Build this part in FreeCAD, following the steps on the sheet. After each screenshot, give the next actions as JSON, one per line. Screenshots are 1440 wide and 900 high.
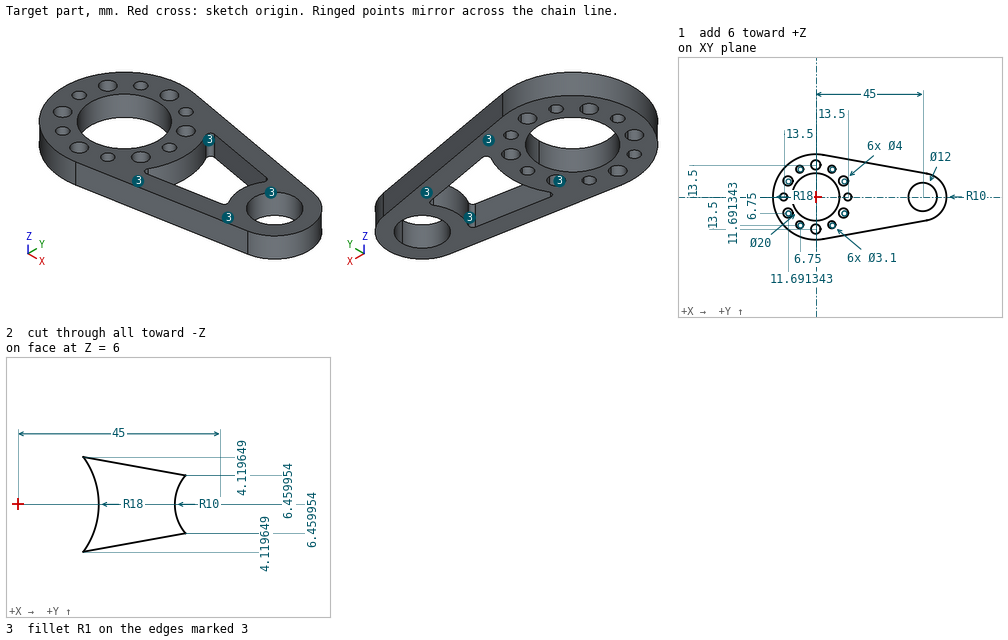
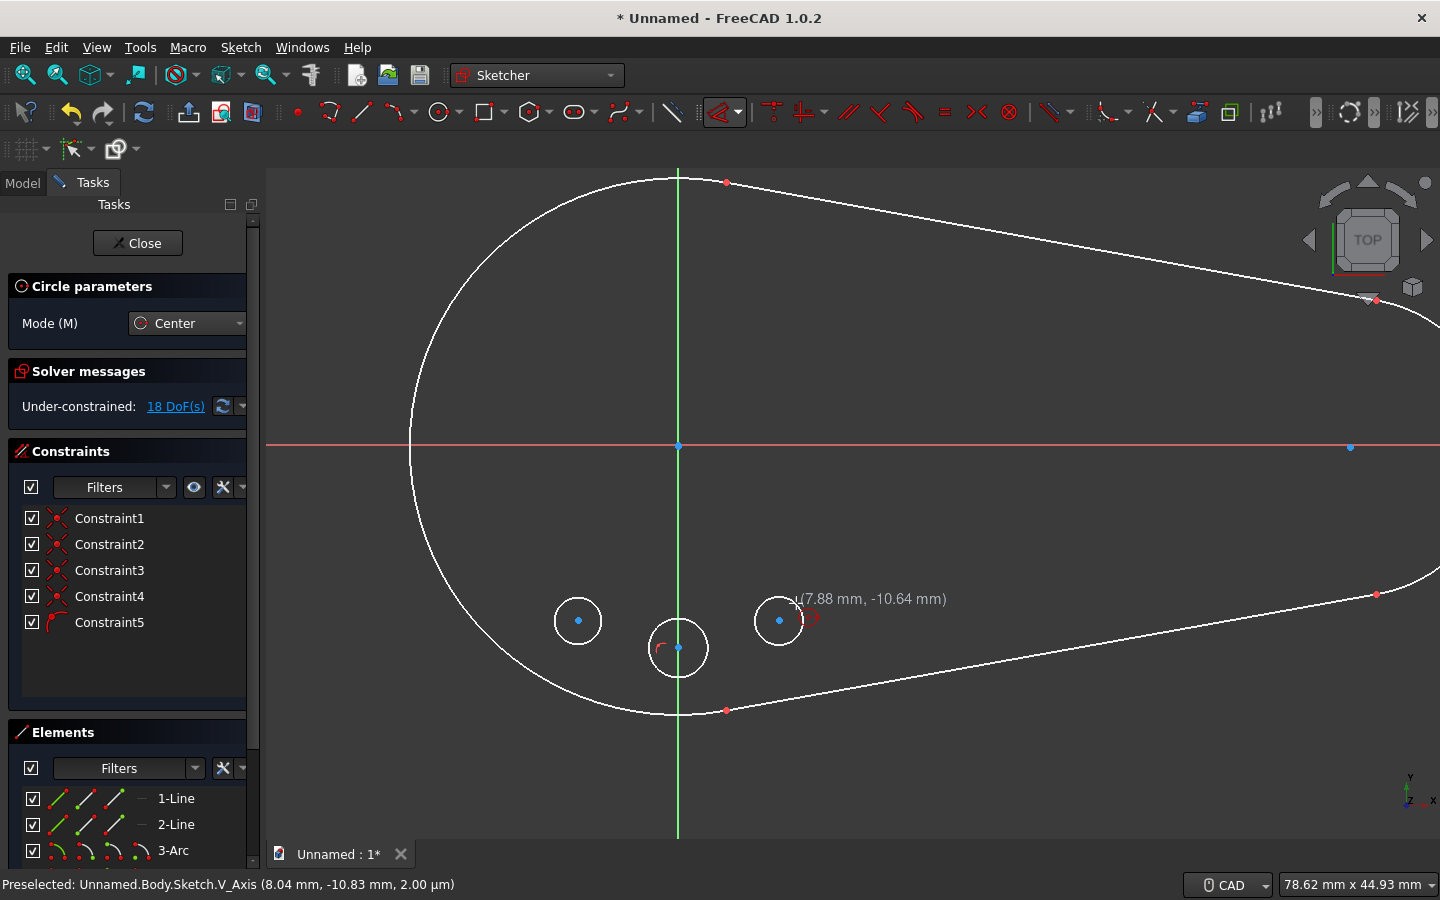
{"action": "left_click", "coordinate": [504, 546]}
{"action": "left_click", "coordinate": [525, 525]}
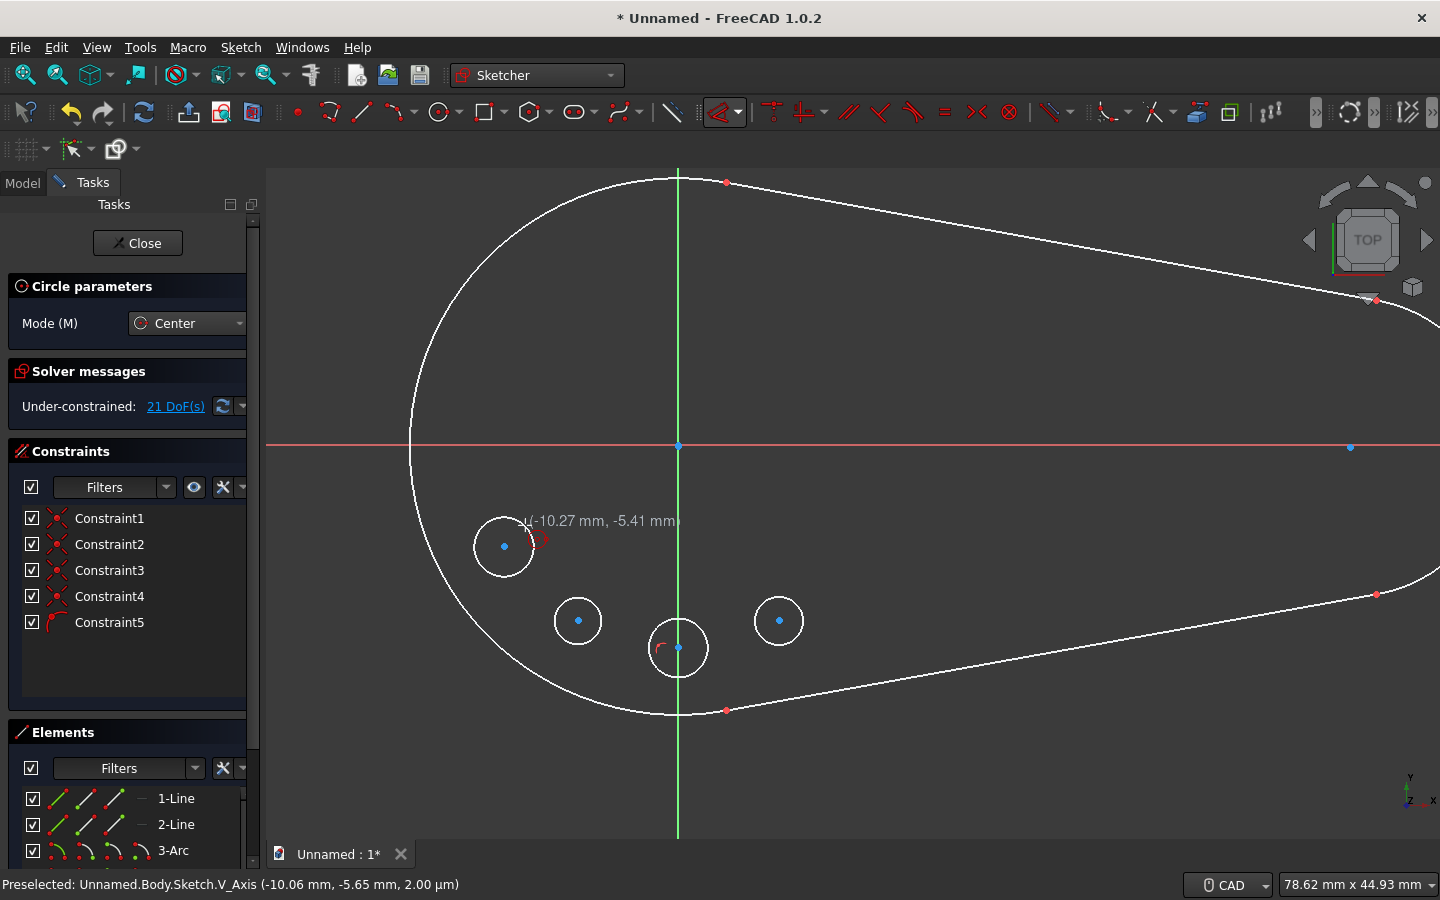
{"action": "left_click", "coordinate": [853, 546]}
{"action": "left_click", "coordinate": [874, 525]}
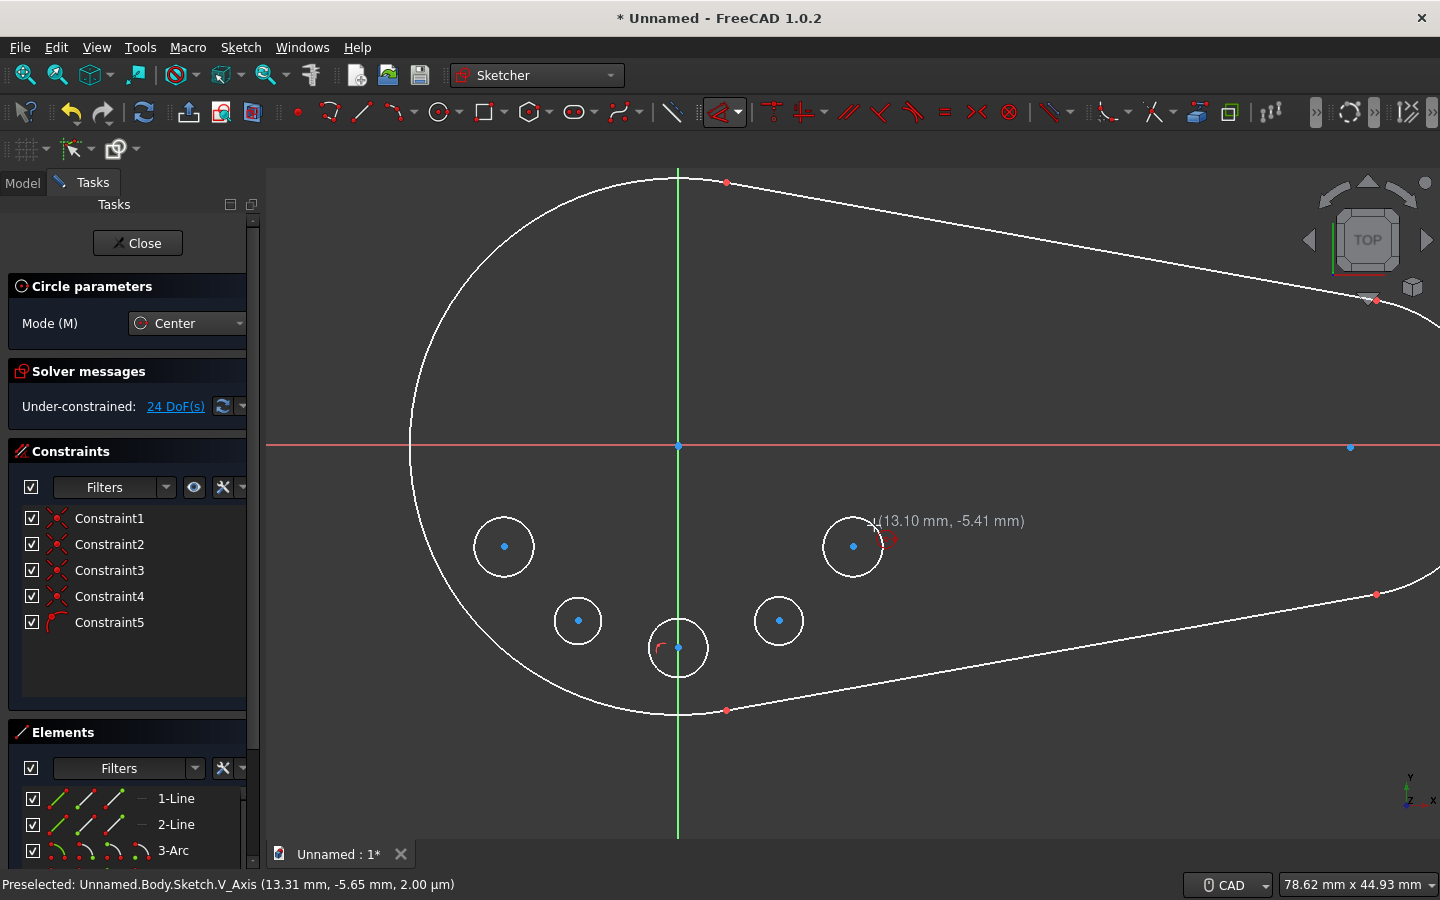
{"action": "left_click", "coordinate": [477, 445]}
{"action": "left_click", "coordinate": [493, 429]}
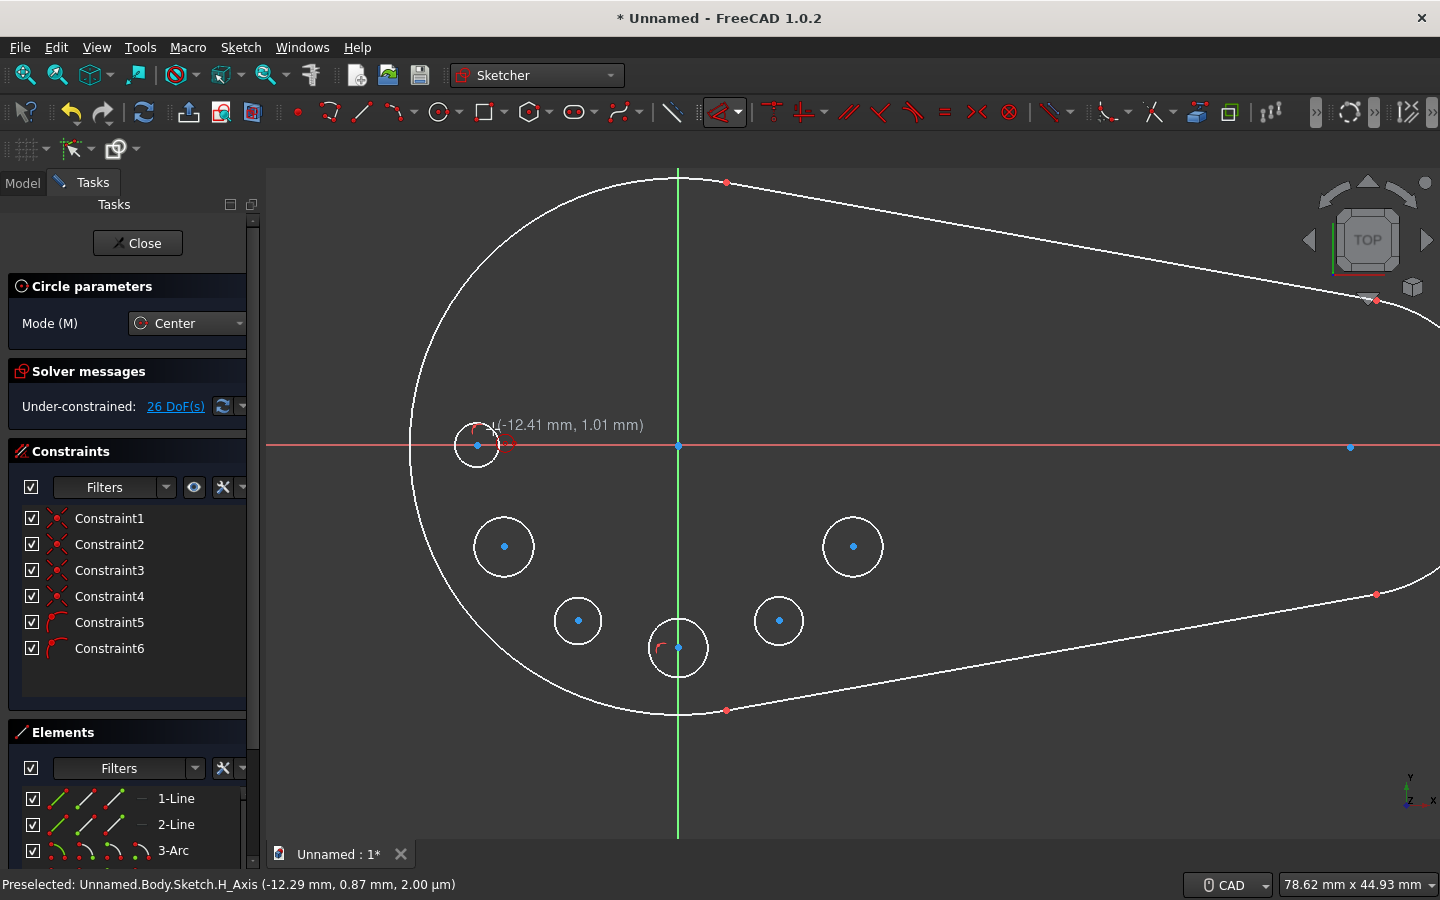
{"action": "left_click", "coordinate": [678, 445]}
{"action": "left_click", "coordinate": [784, 340]}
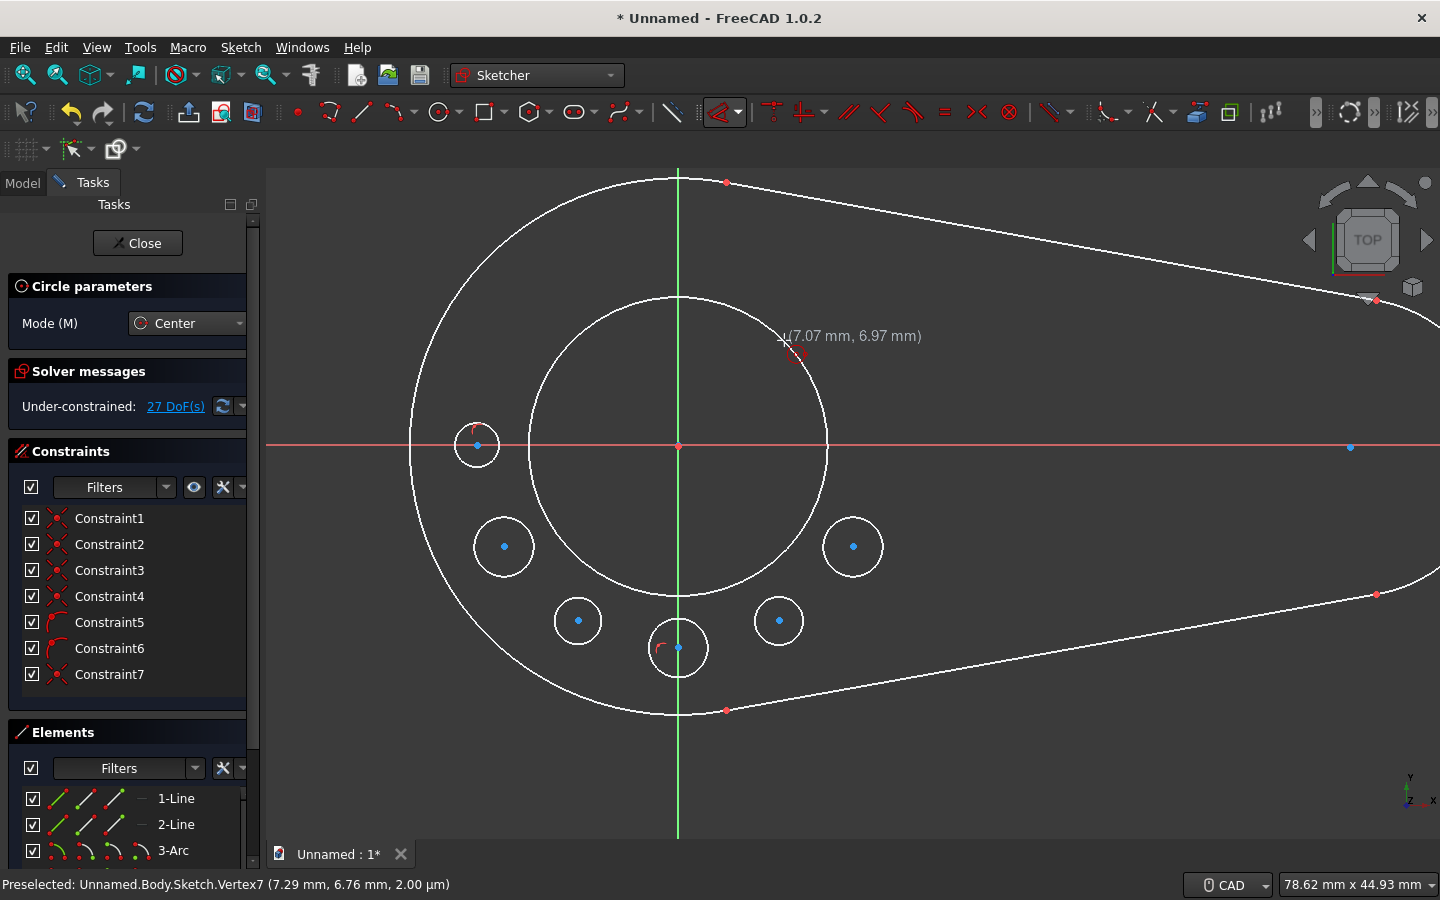
{"action": "left_click", "coordinate": [504, 344]}
{"action": "left_click", "coordinate": [525, 323]}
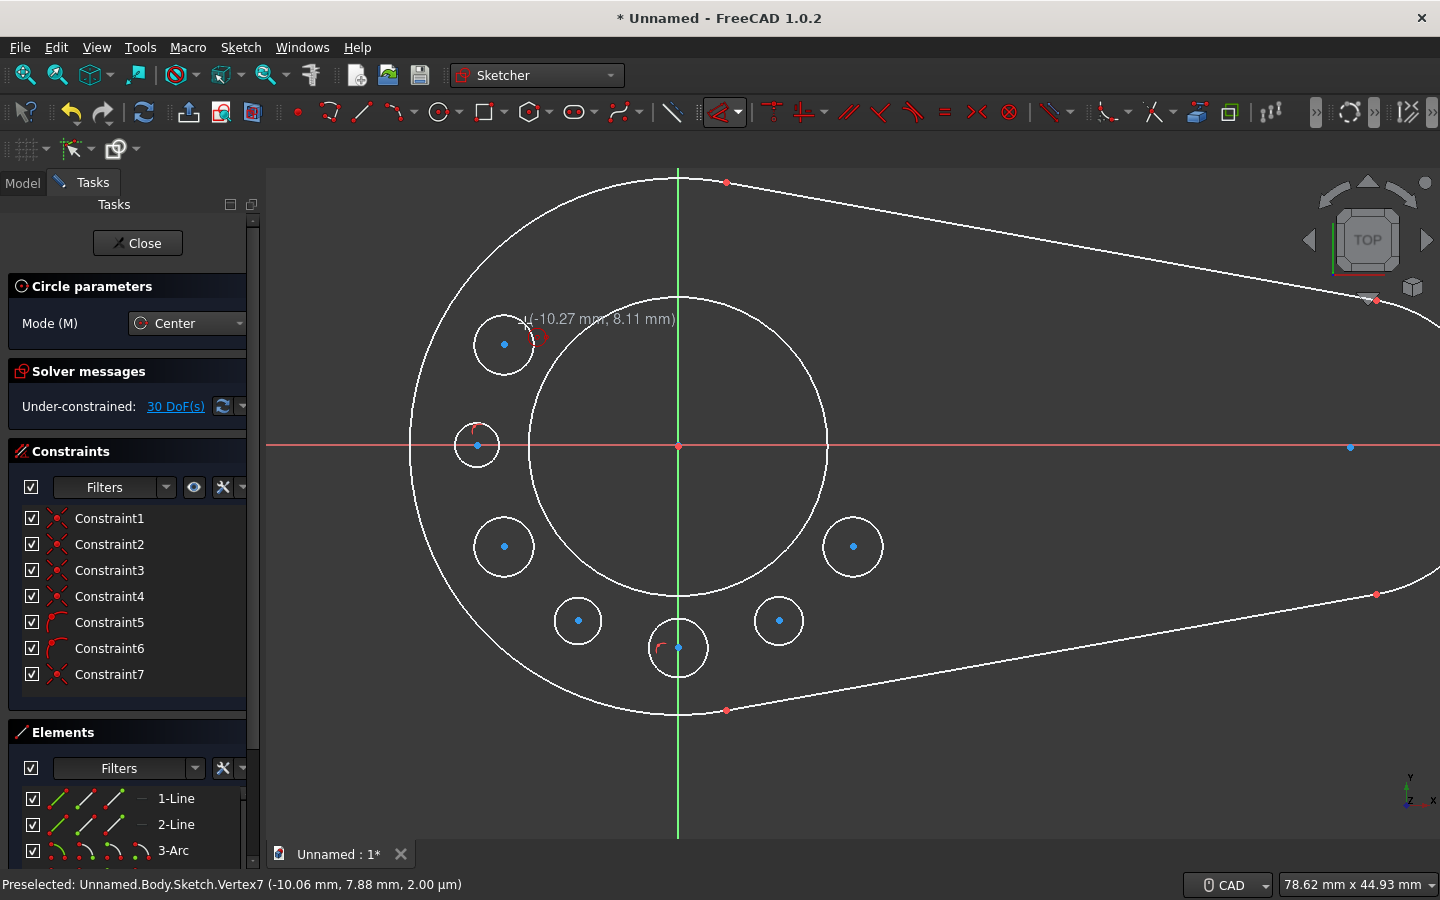
{"action": "left_click", "coordinate": [880, 445]}
{"action": "left_click", "coordinate": [896, 429]}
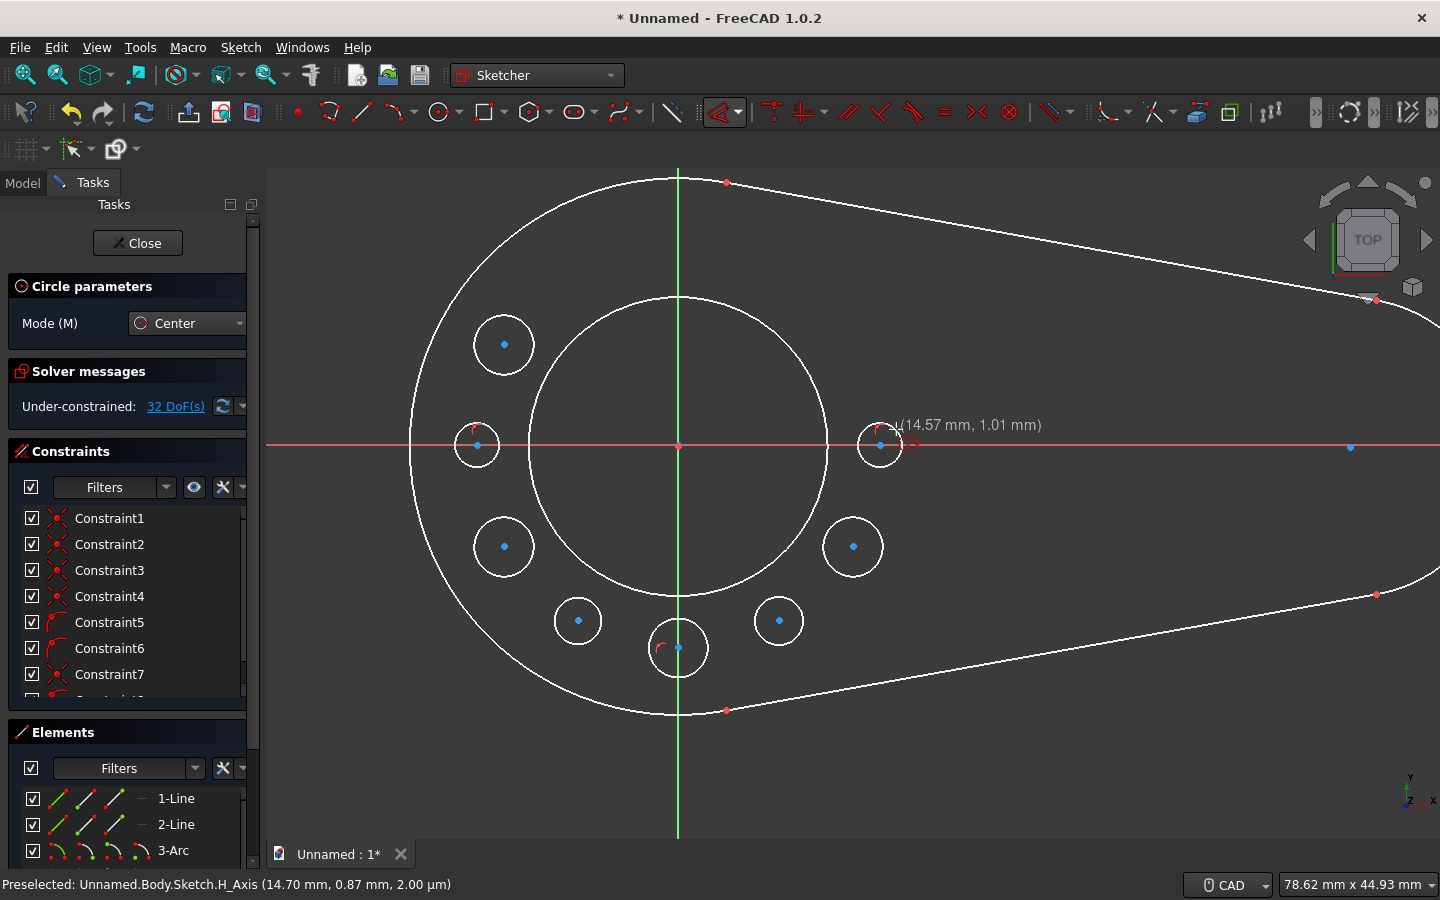
{"action": "left_click", "coordinate": [853, 344]}
{"action": "left_click", "coordinate": [874, 323]}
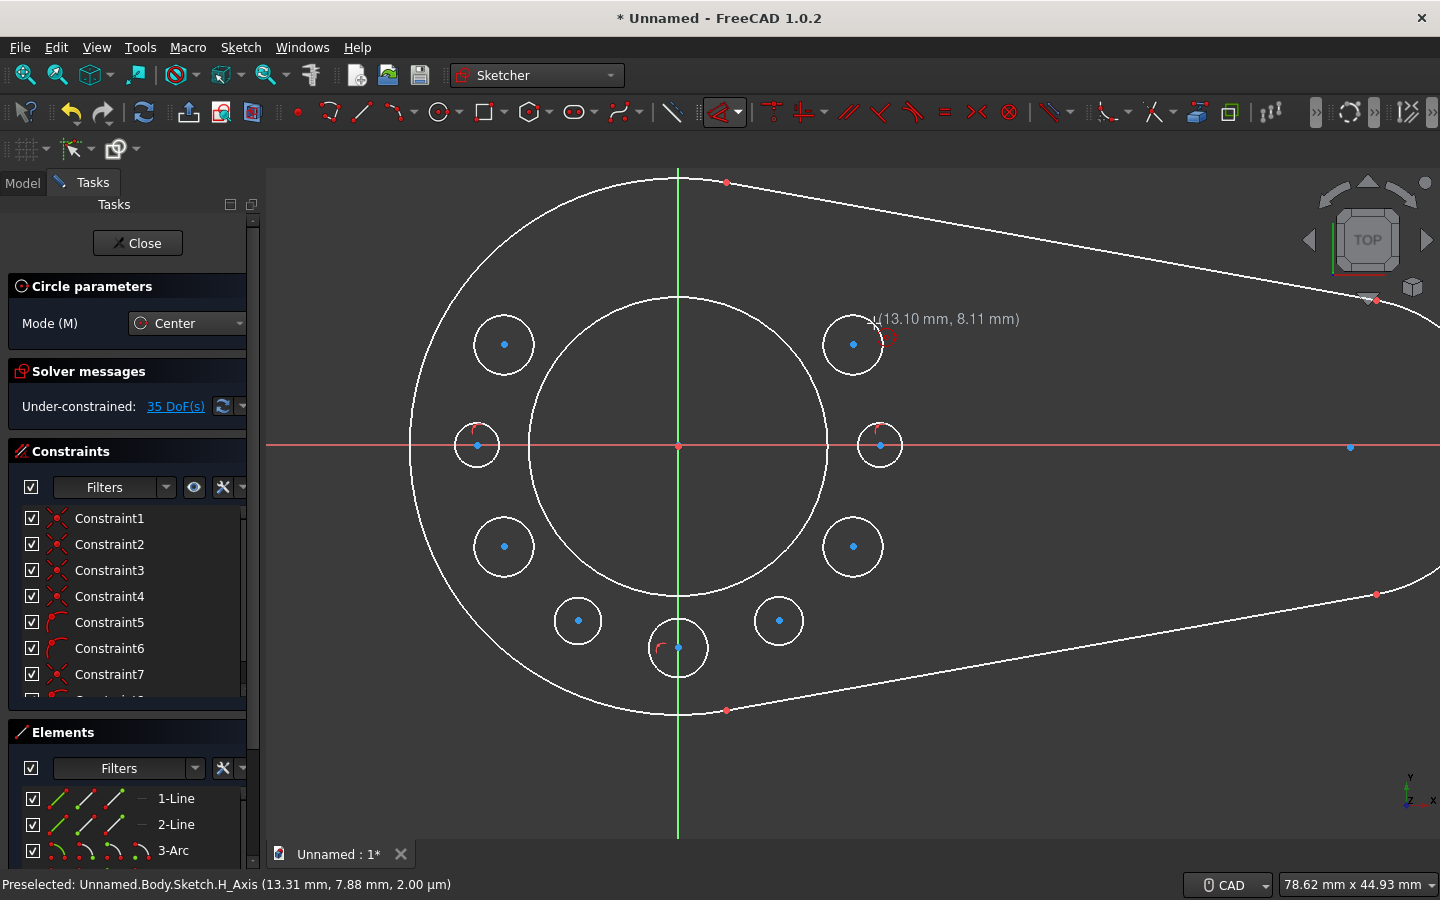
{"action": "left_click", "coordinate": [578, 271]}
{"action": "left_click", "coordinate": [594, 254]}